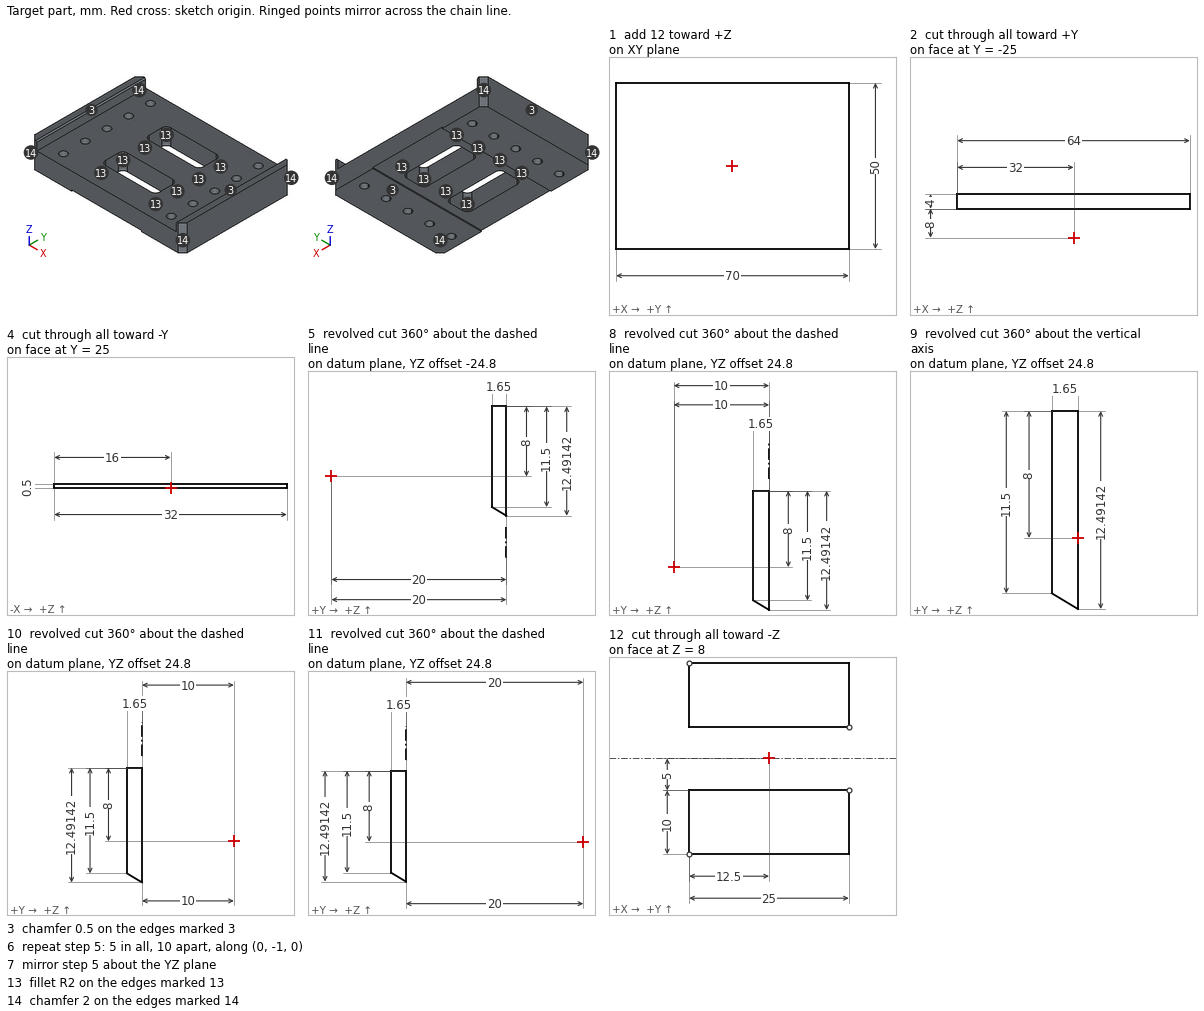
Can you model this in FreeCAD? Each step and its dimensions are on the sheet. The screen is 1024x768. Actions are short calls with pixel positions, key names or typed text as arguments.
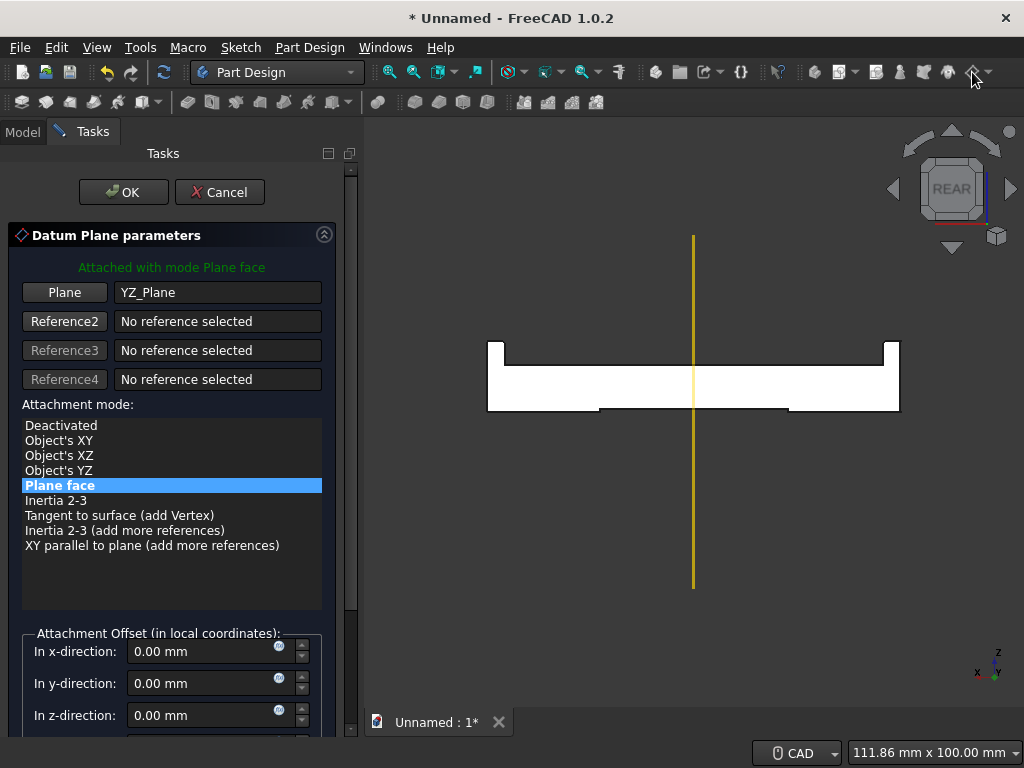
triple_click(210, 715)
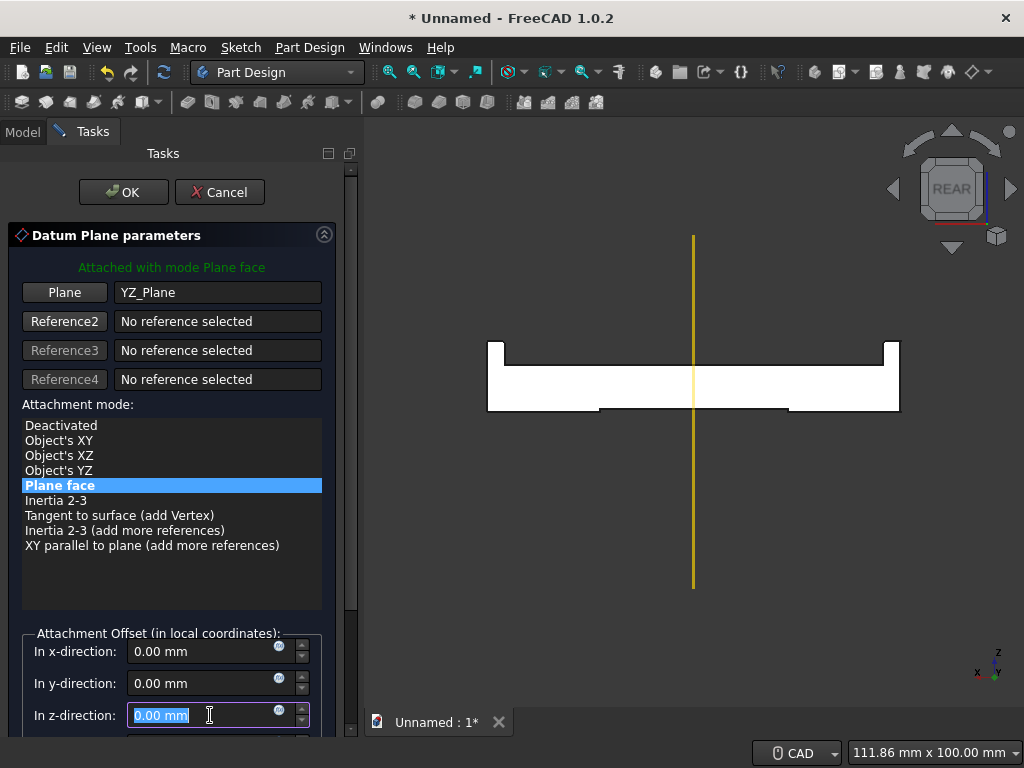
text(-24.8)
key(Tab)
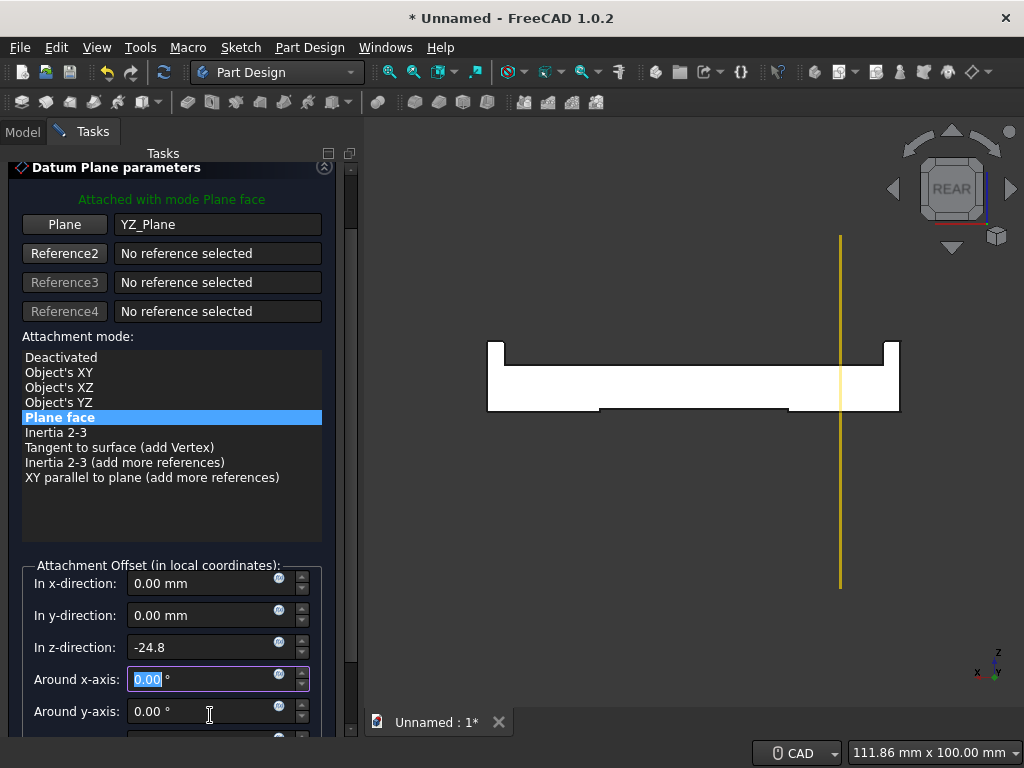
scroll(351, 450, up, 2)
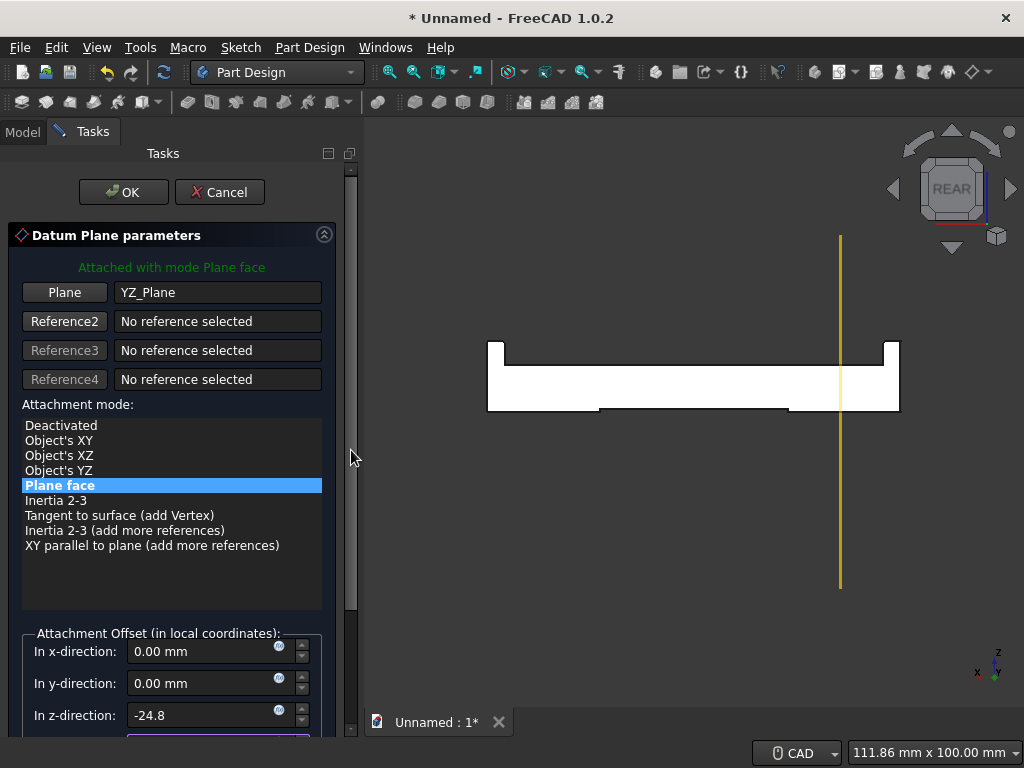
click(124, 192)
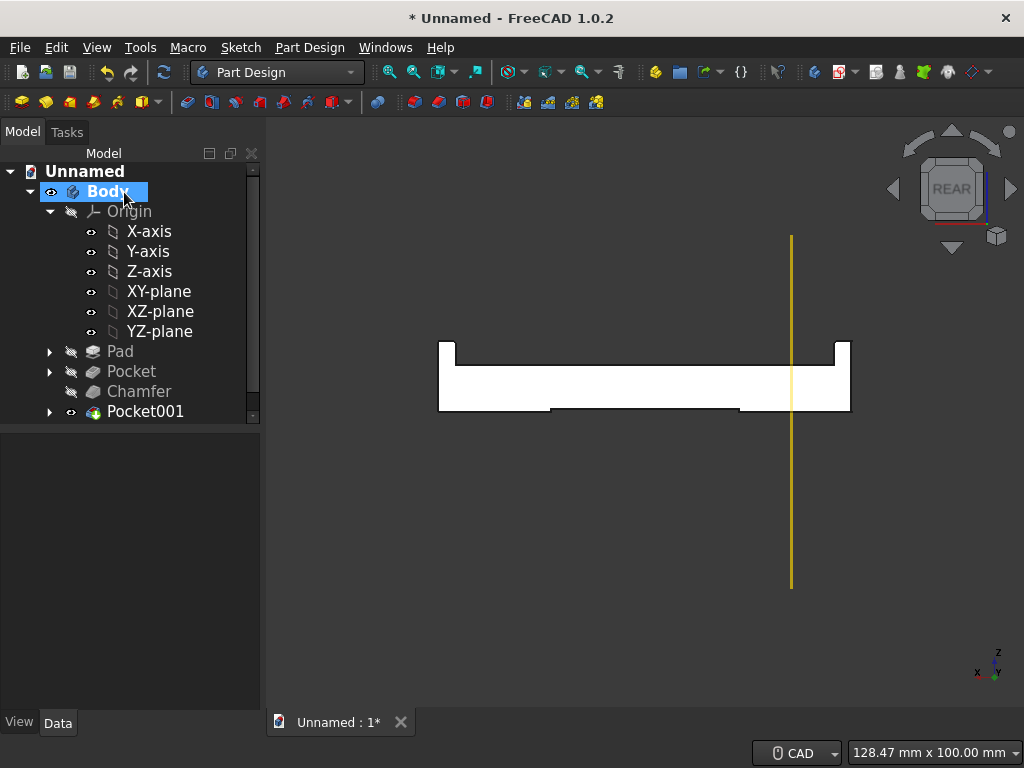
scroll(100, 287, down, 3)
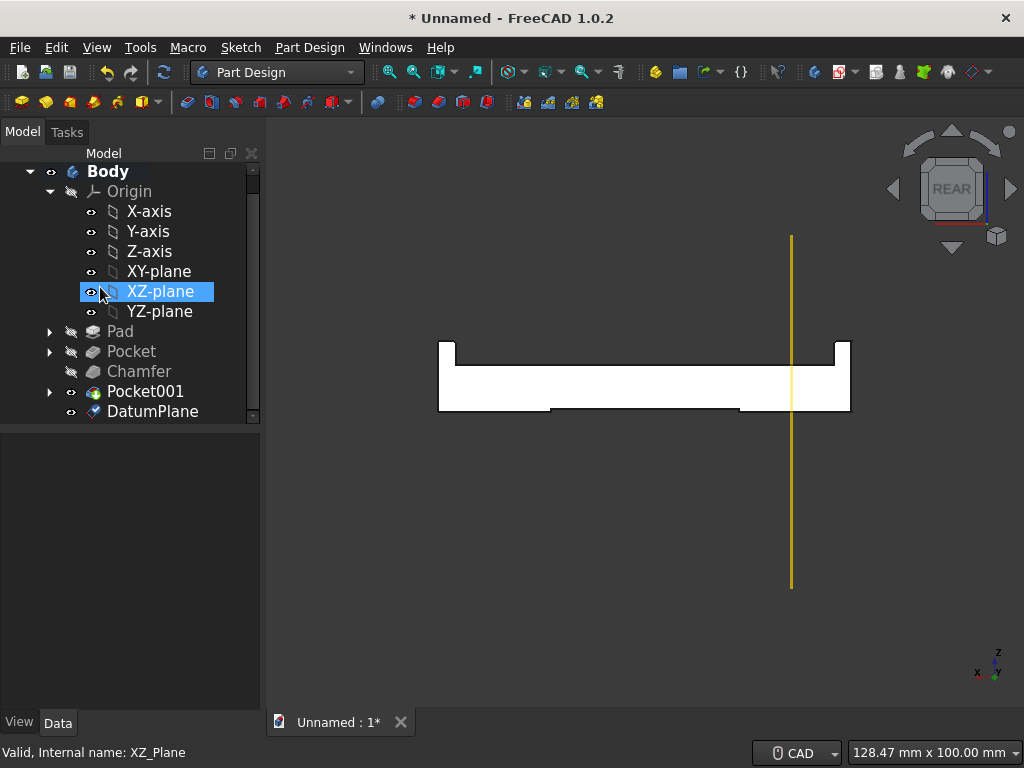
click(116, 412)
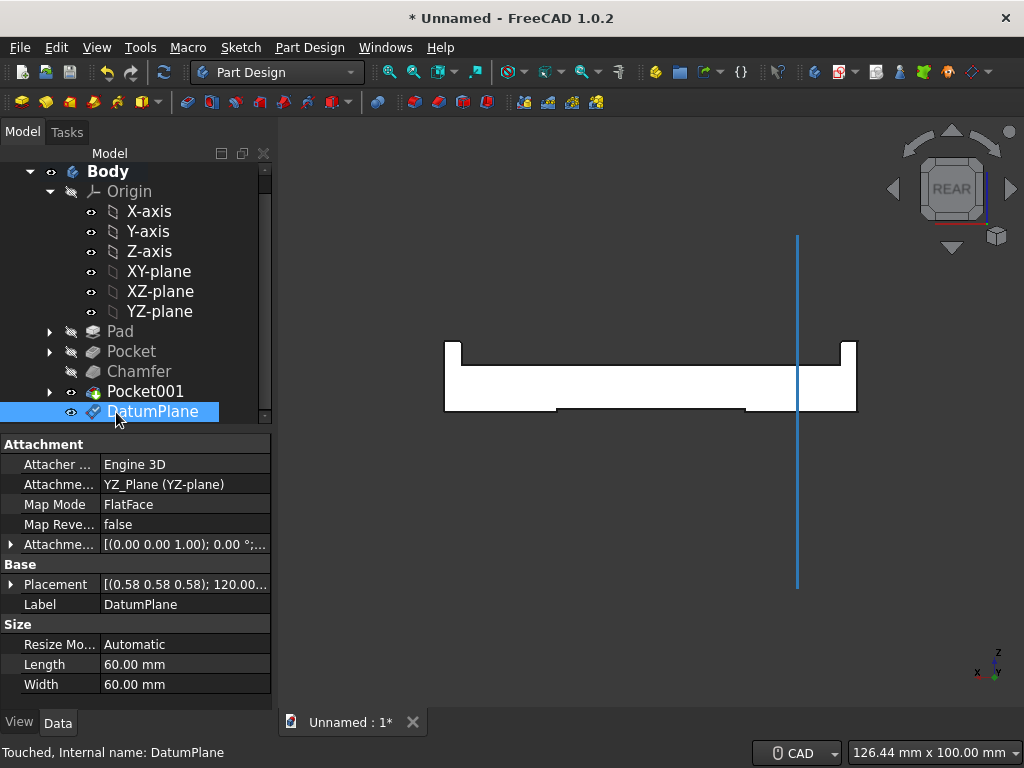
click(840, 72)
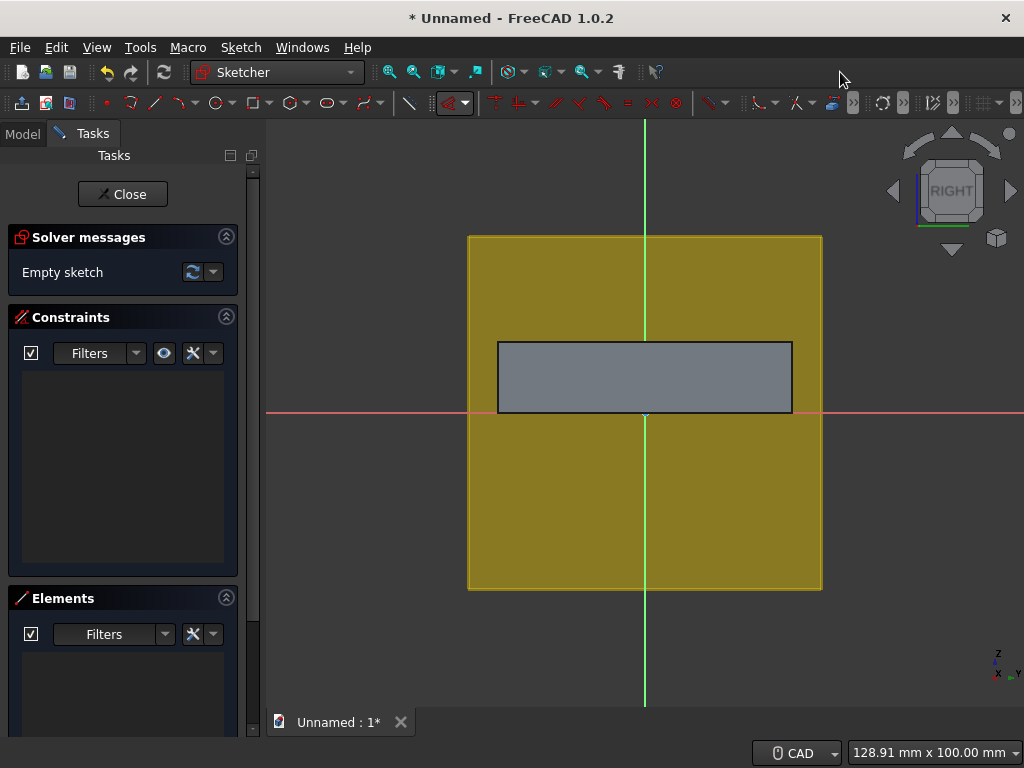
key(q)
key(s)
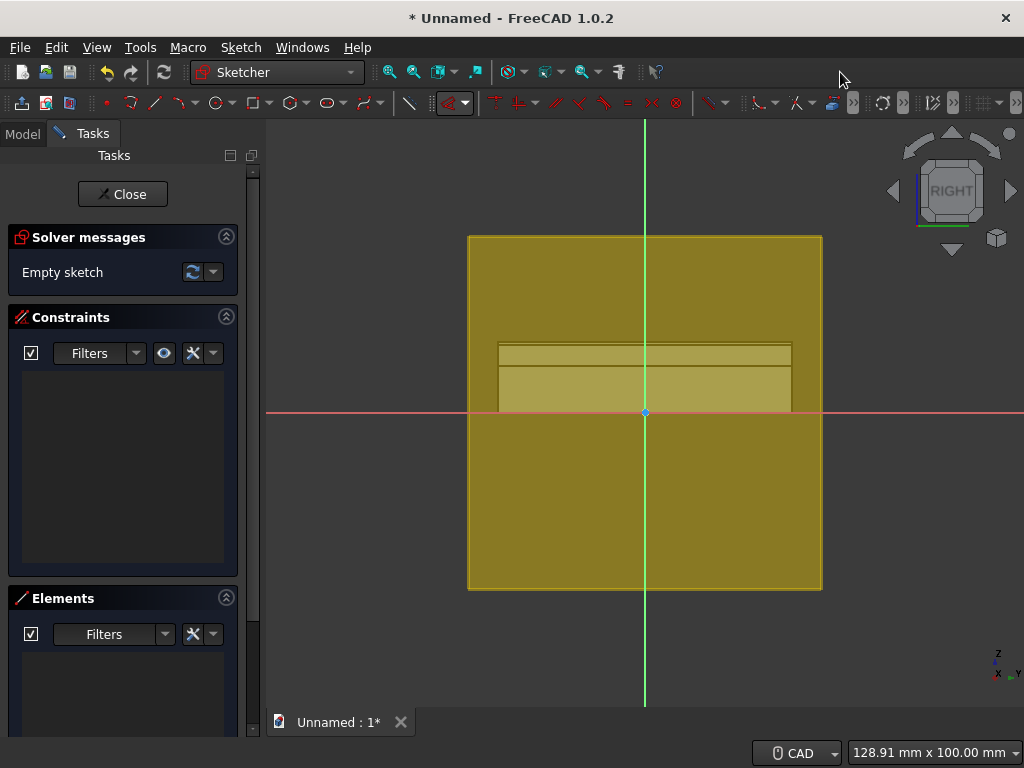
scroll(759, 419, up, 6)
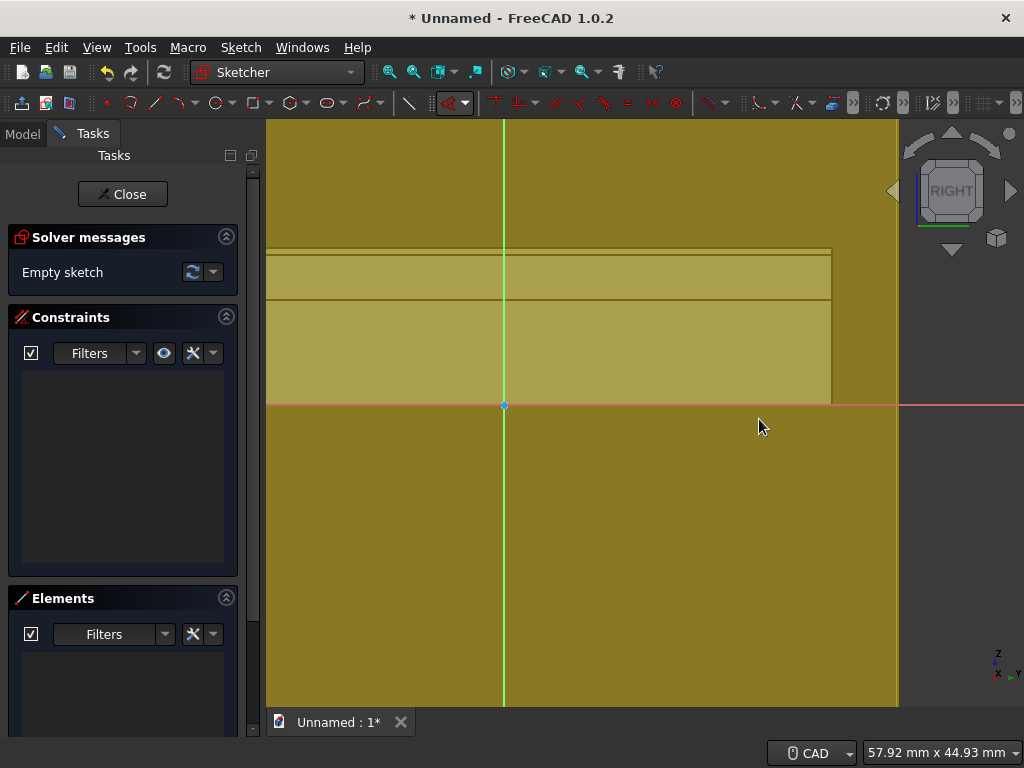
key(g)
key(m)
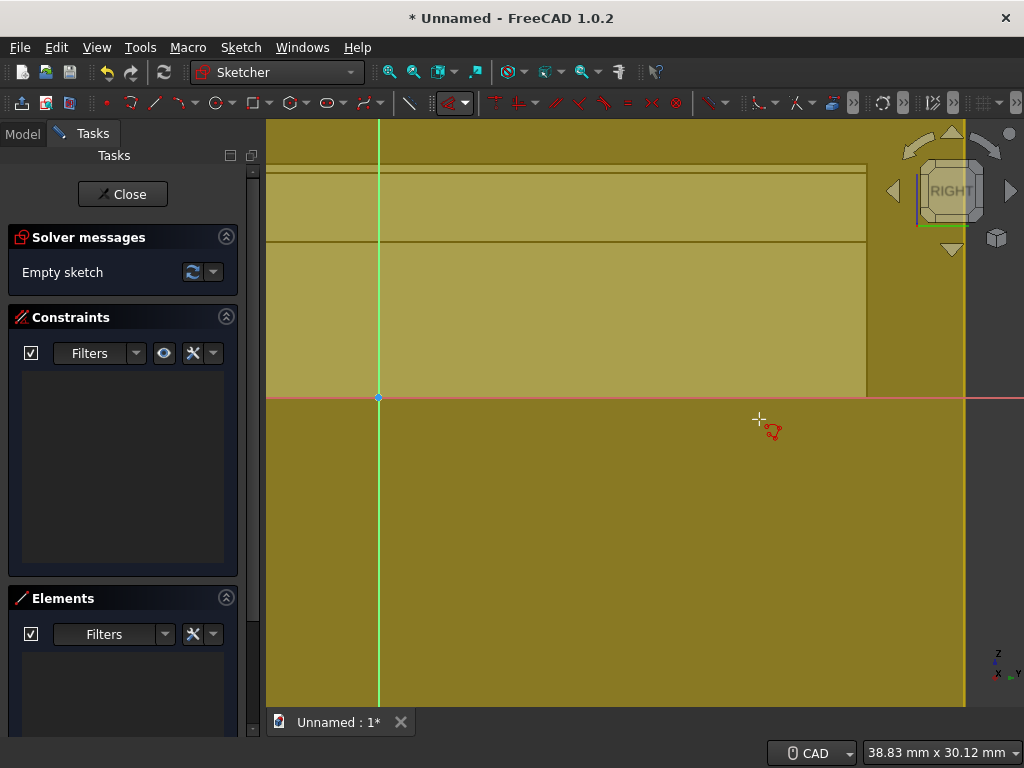
click(737, 466)
click(769, 486)
click(769, 242)
click(737, 242)
click(737, 467)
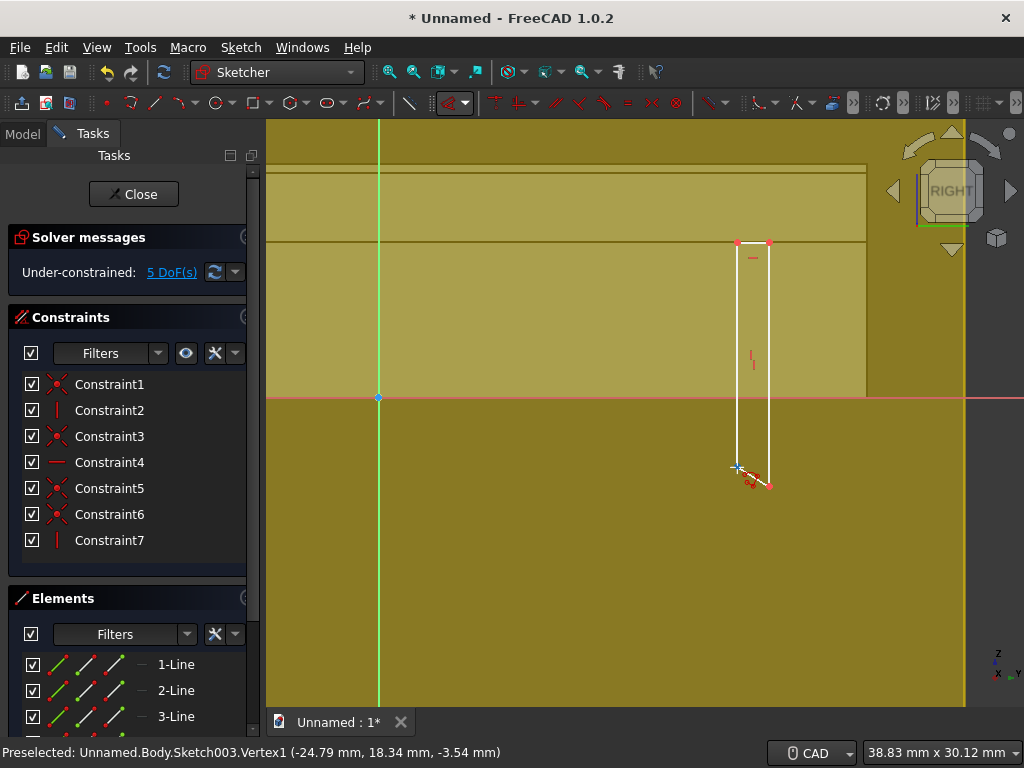
click(156, 104)